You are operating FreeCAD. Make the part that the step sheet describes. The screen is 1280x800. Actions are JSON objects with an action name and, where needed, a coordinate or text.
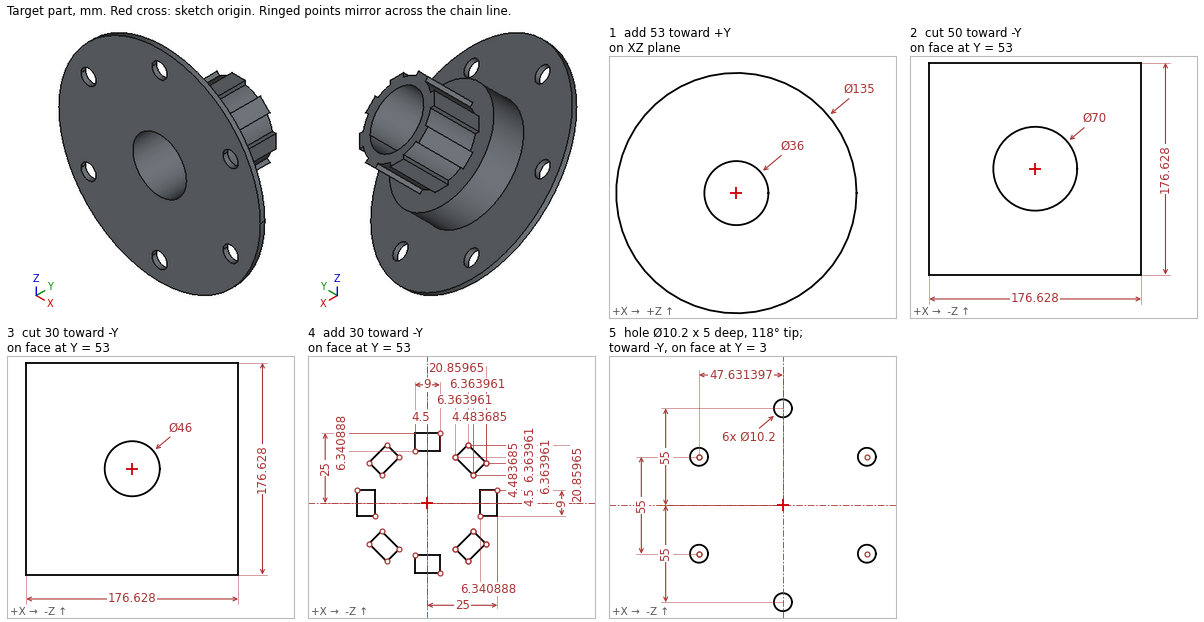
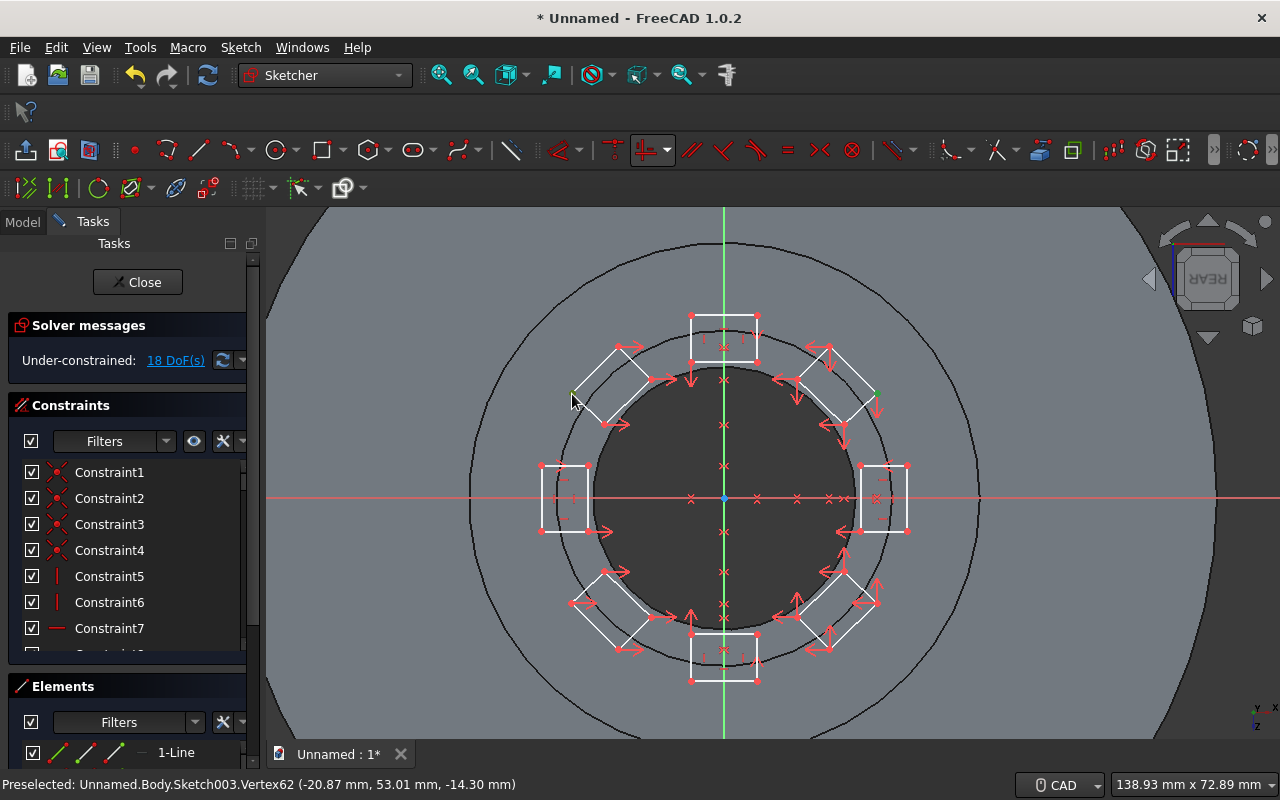
{"action": "left_click", "coordinate": [724, 541]}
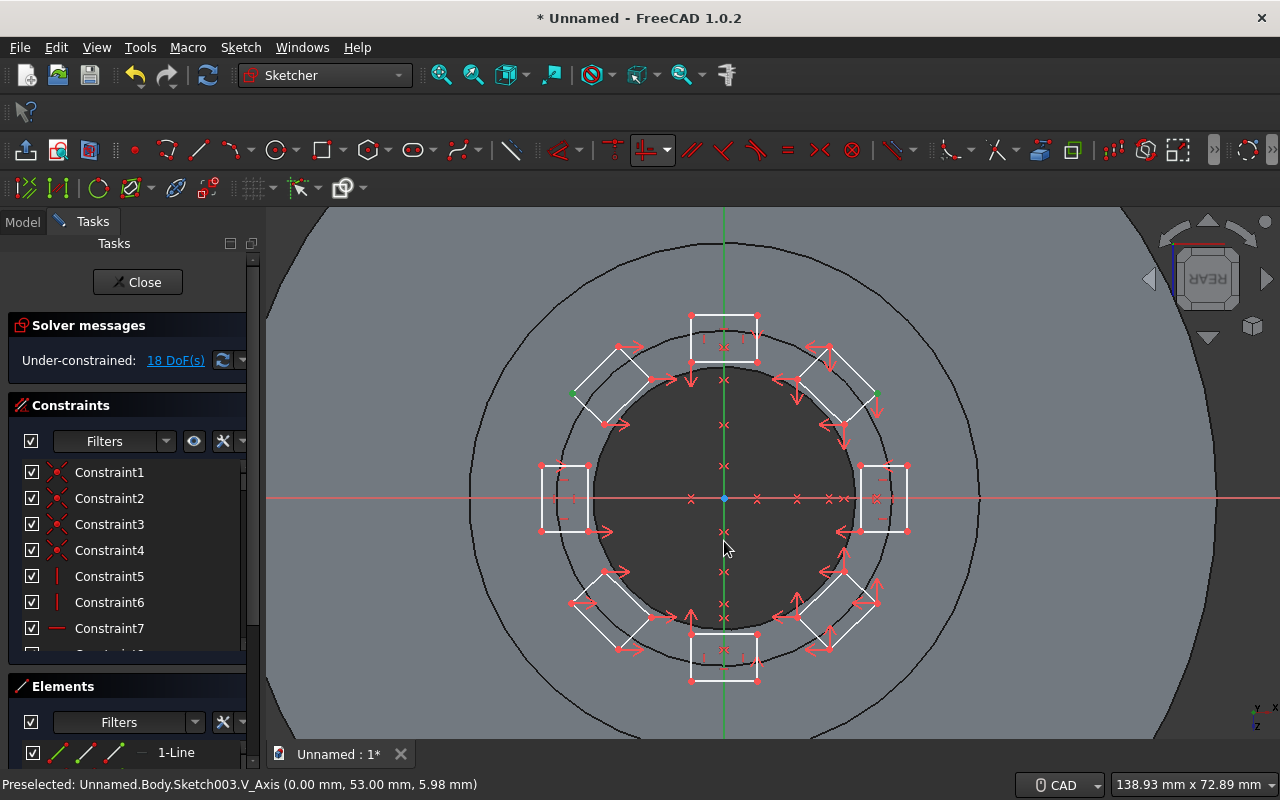
{"action": "left_click", "coordinate": [820, 150]}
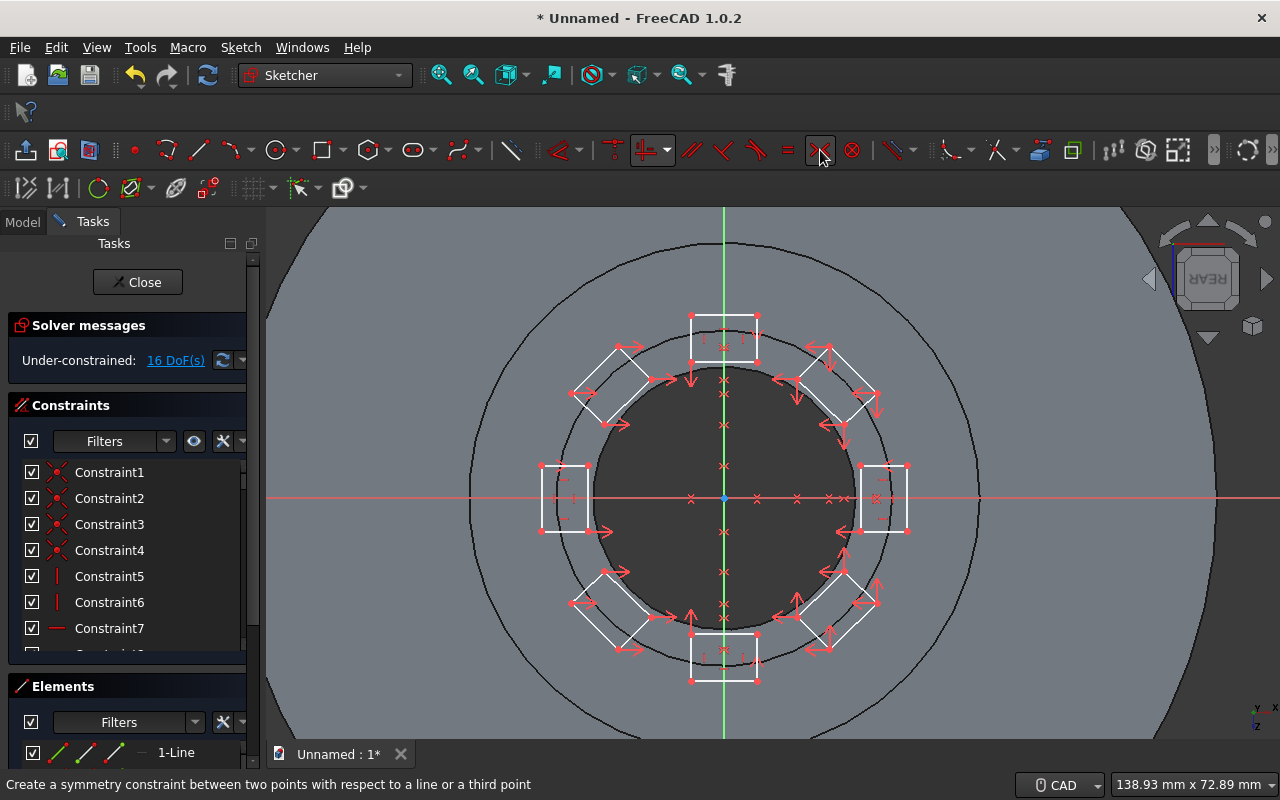
{"action": "left_click", "coordinate": [558, 150]}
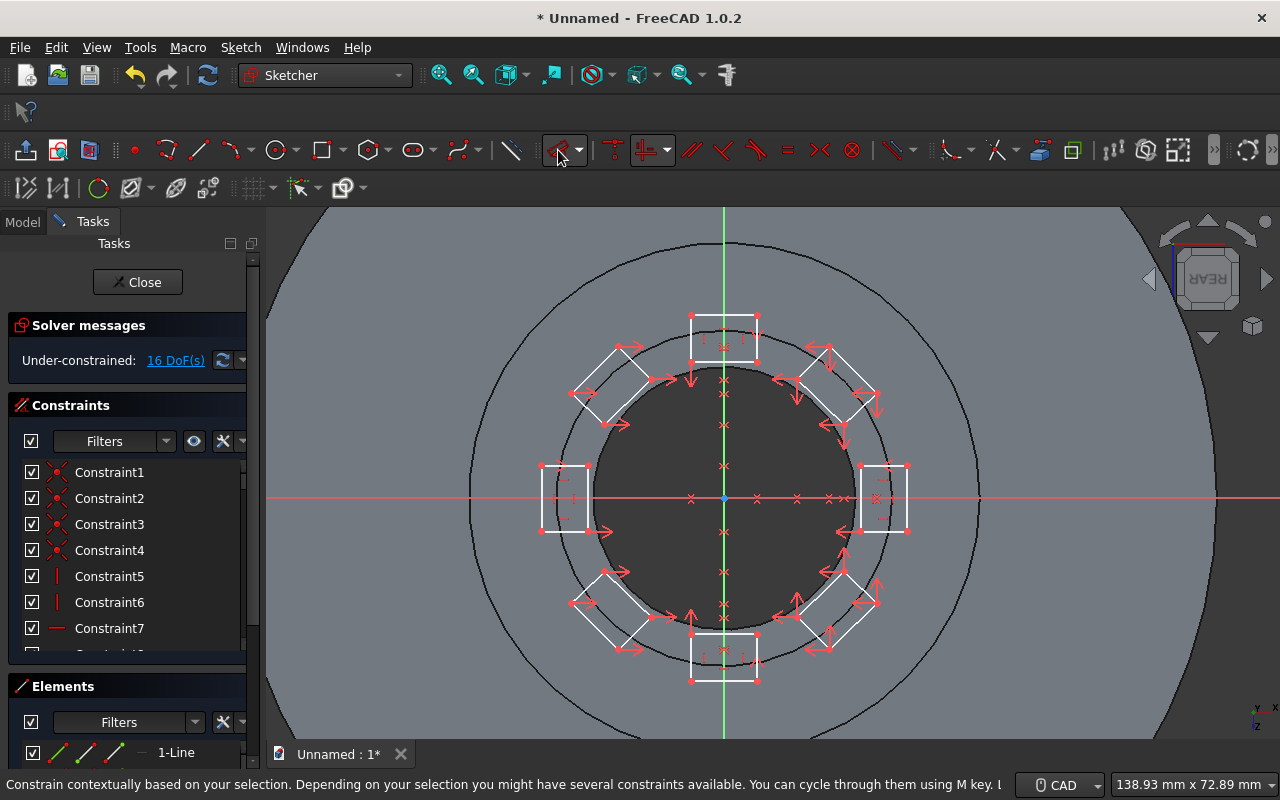
{"action": "left_click", "coordinate": [711, 362]}
{"action": "left_click", "coordinate": [709, 328]}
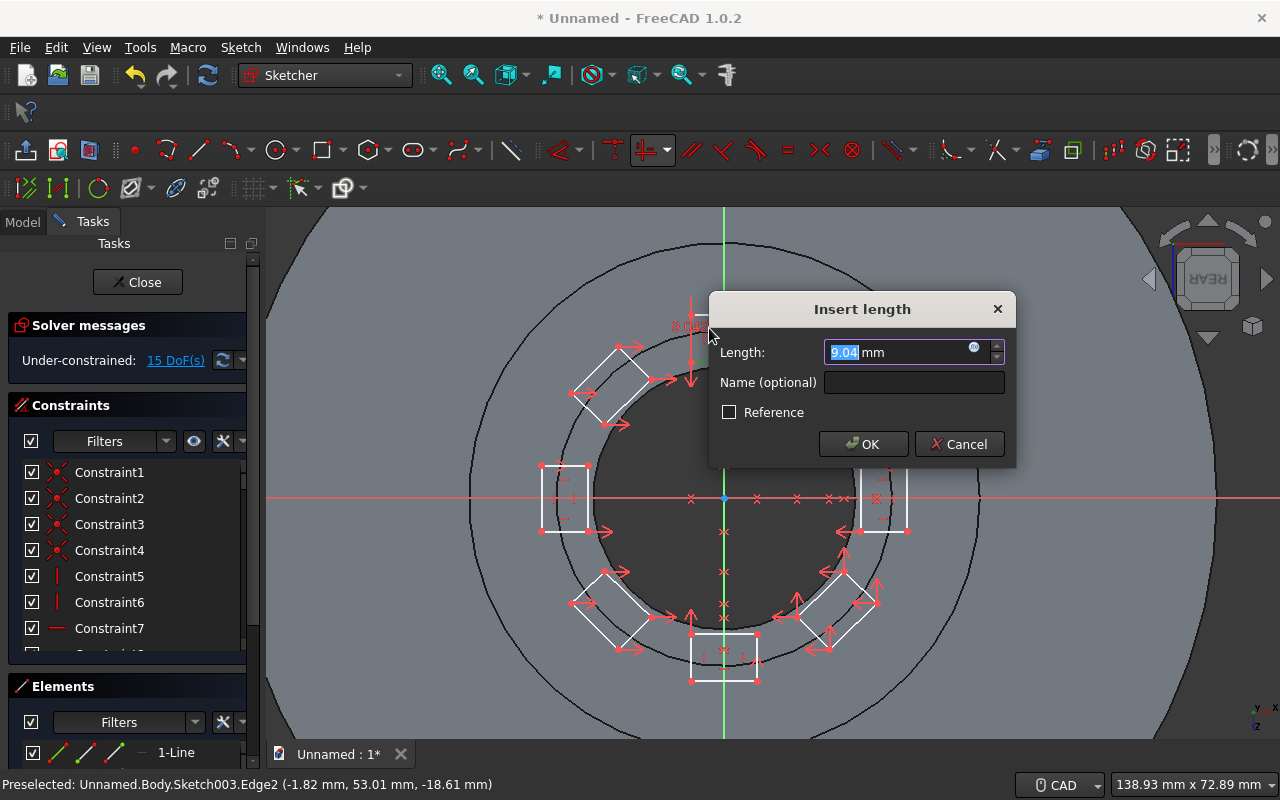
{"action": "type", "text": "9"}
{"action": "key", "text": "Return"}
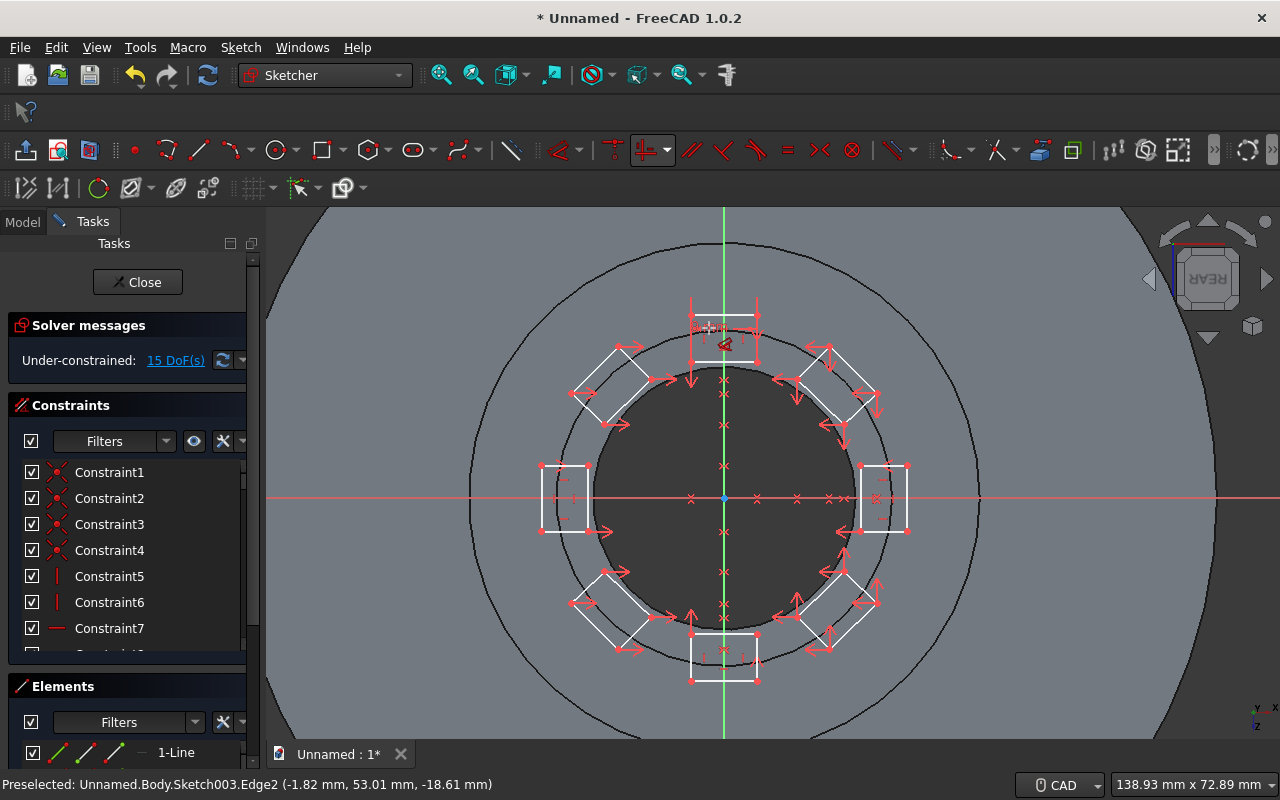
{"action": "left_click", "coordinate": [861, 486]}
{"action": "left_click", "coordinate": [827, 484]}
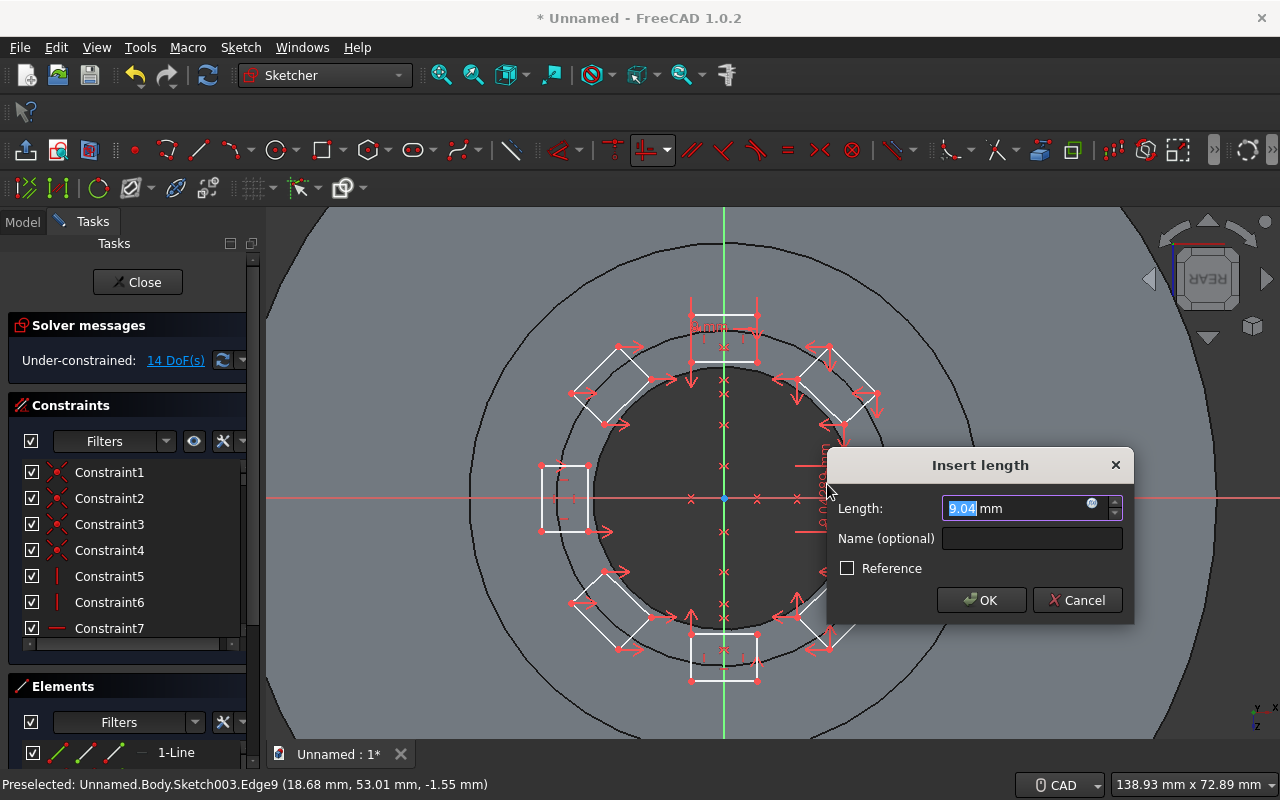
{"action": "type", "text": "9"}
{"action": "key", "text": "Return"}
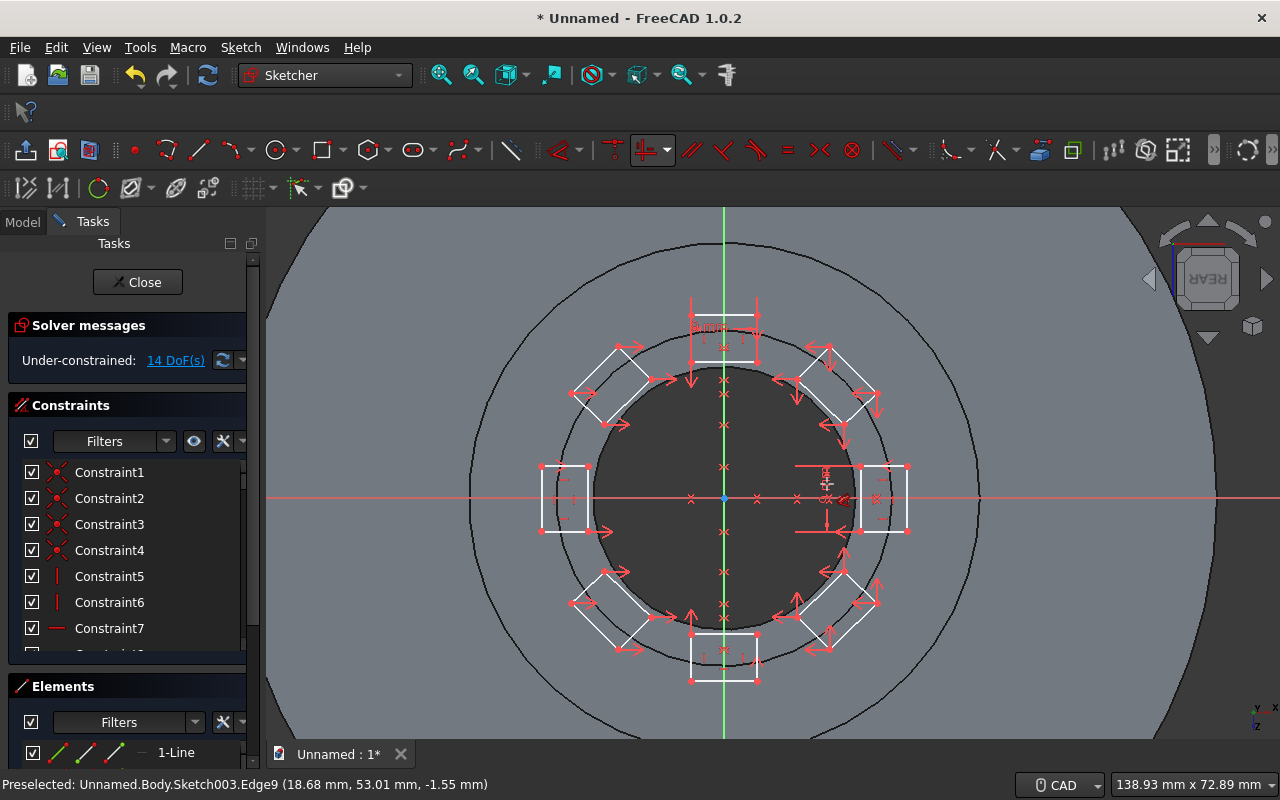
{"action": "left_click", "coordinate": [691, 315]}
{"action": "left_click", "coordinate": [657, 407]}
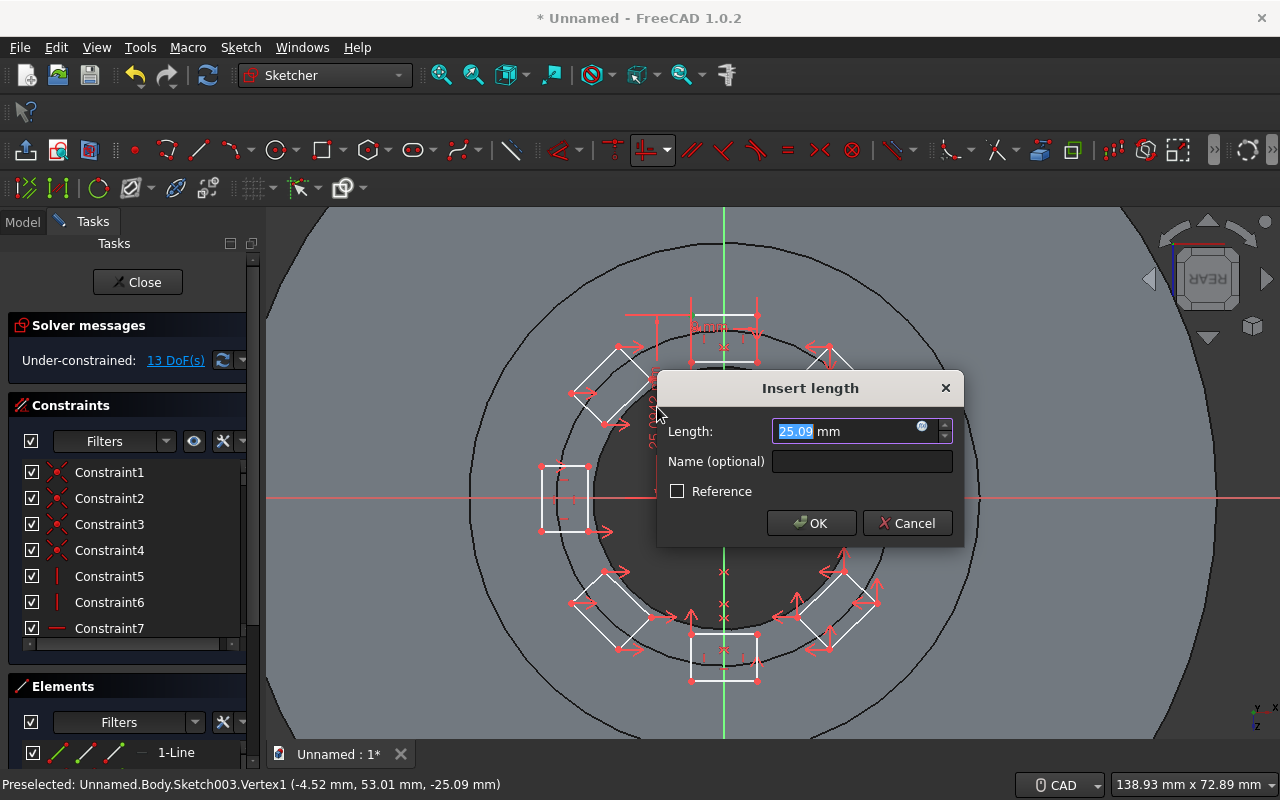
{"action": "type", "text": "25"}
{"action": "key", "text": "Return"}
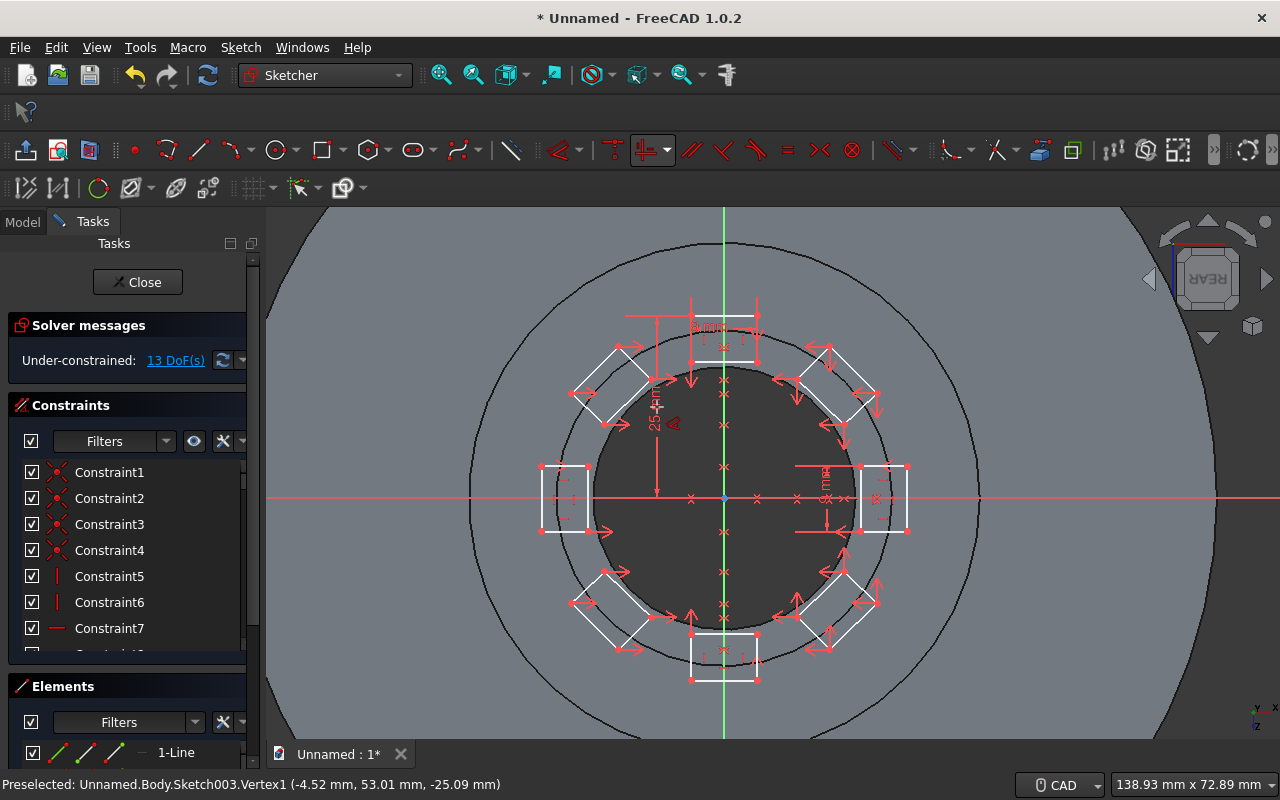
{"action": "left_click", "coordinate": [907, 532]}
{"action": "left_click", "coordinate": [816, 566]}